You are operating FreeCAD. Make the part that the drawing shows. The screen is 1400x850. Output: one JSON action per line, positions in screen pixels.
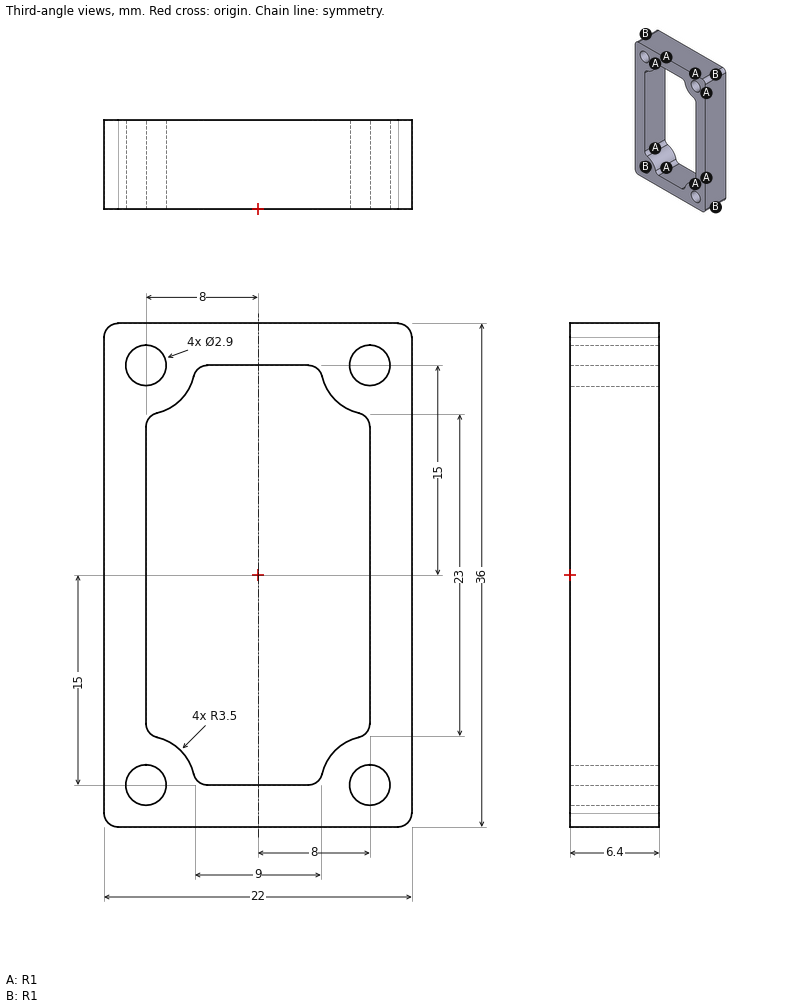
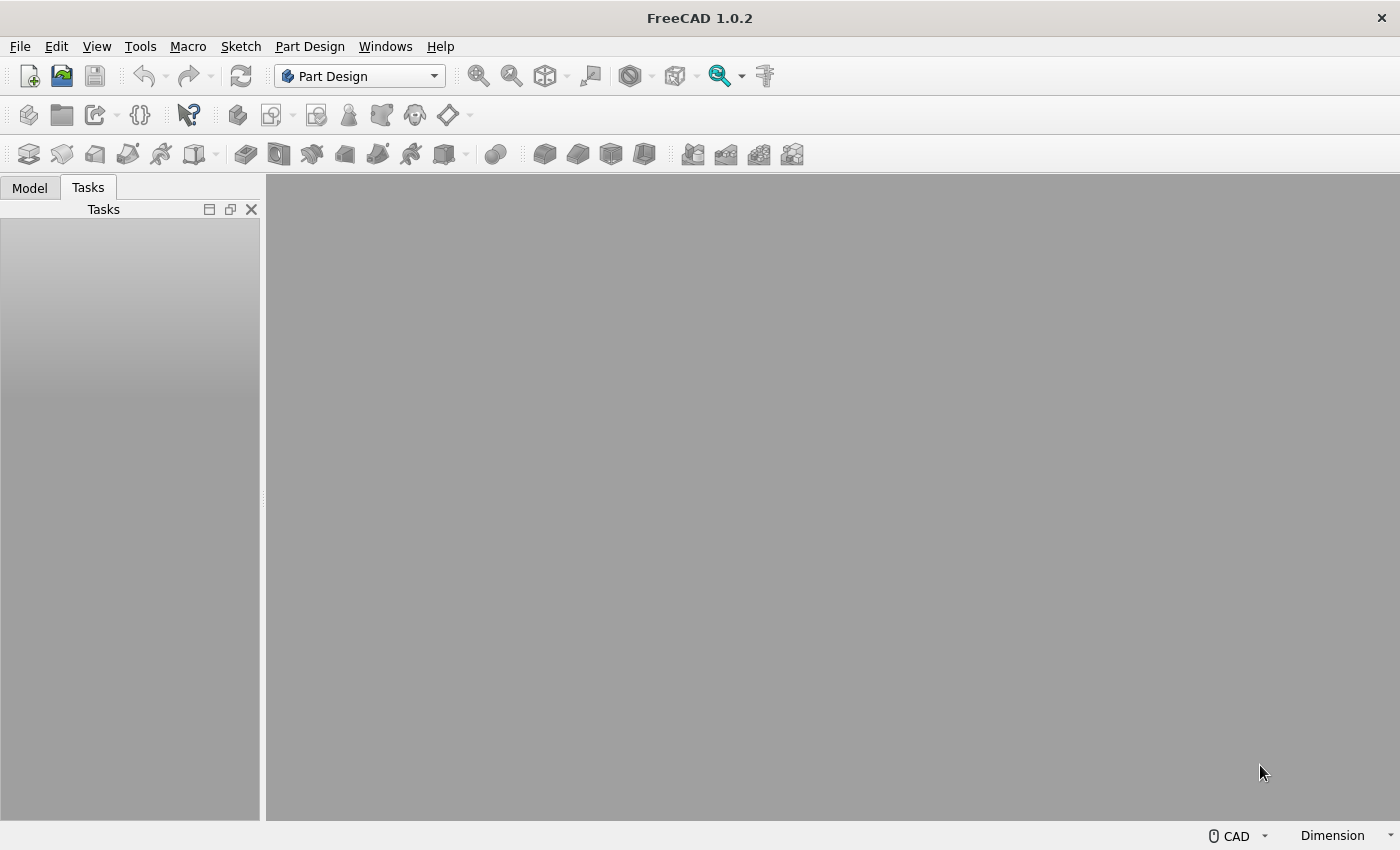
{"action": "left_click", "coordinate": [29, 76]}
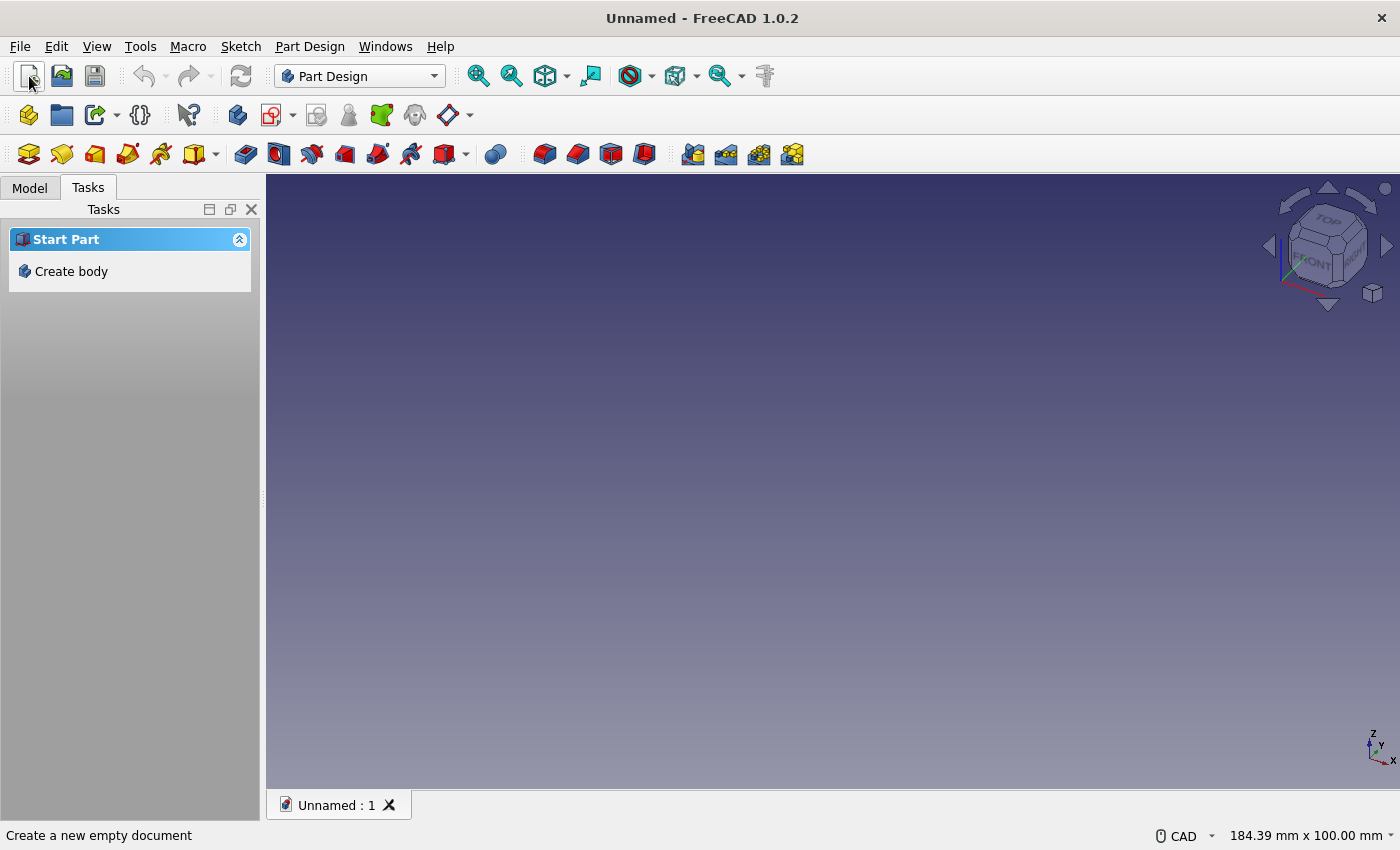
{"action": "left_click", "coordinate": [270, 116]}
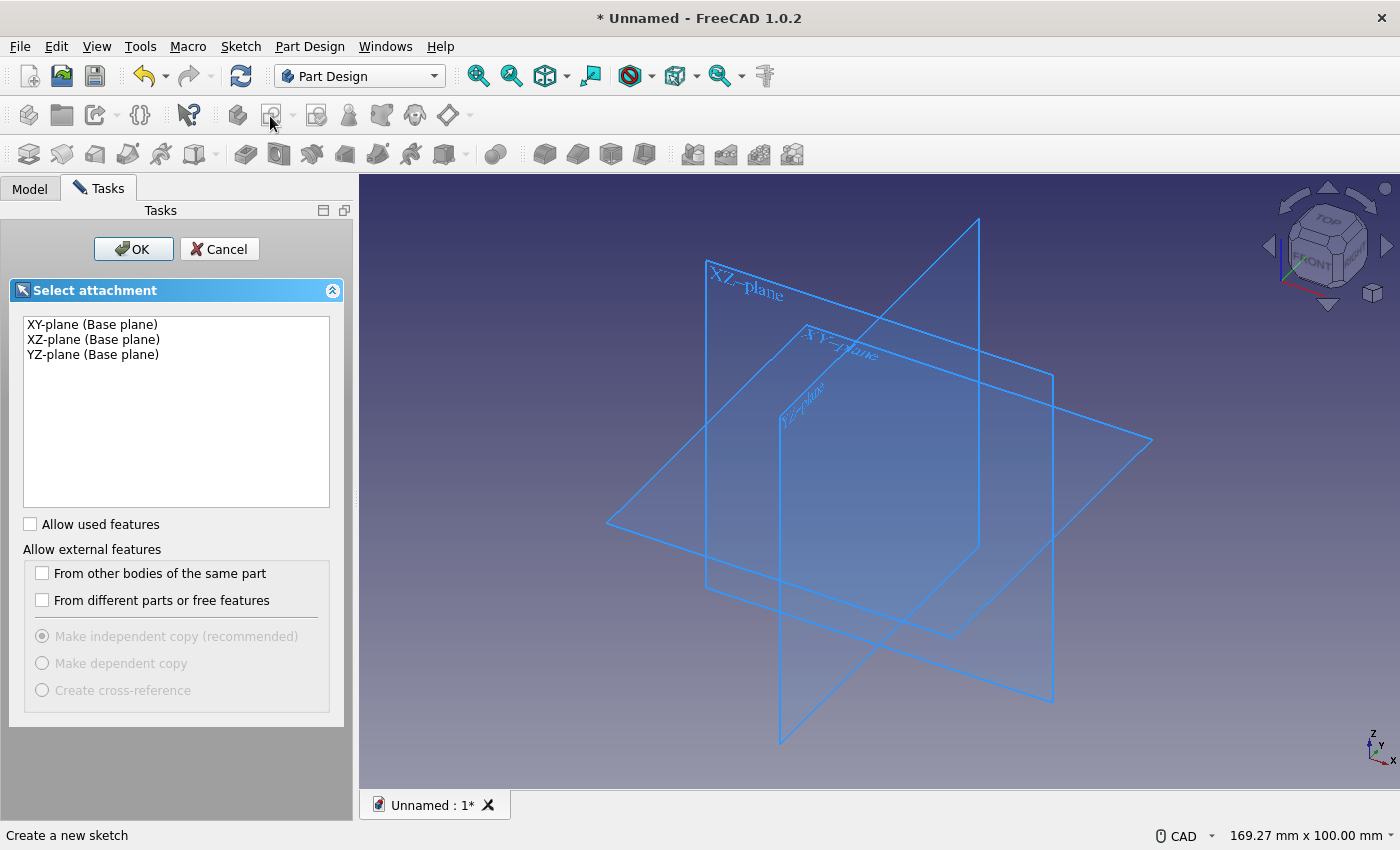
{"action": "left_click", "coordinate": [84, 340]}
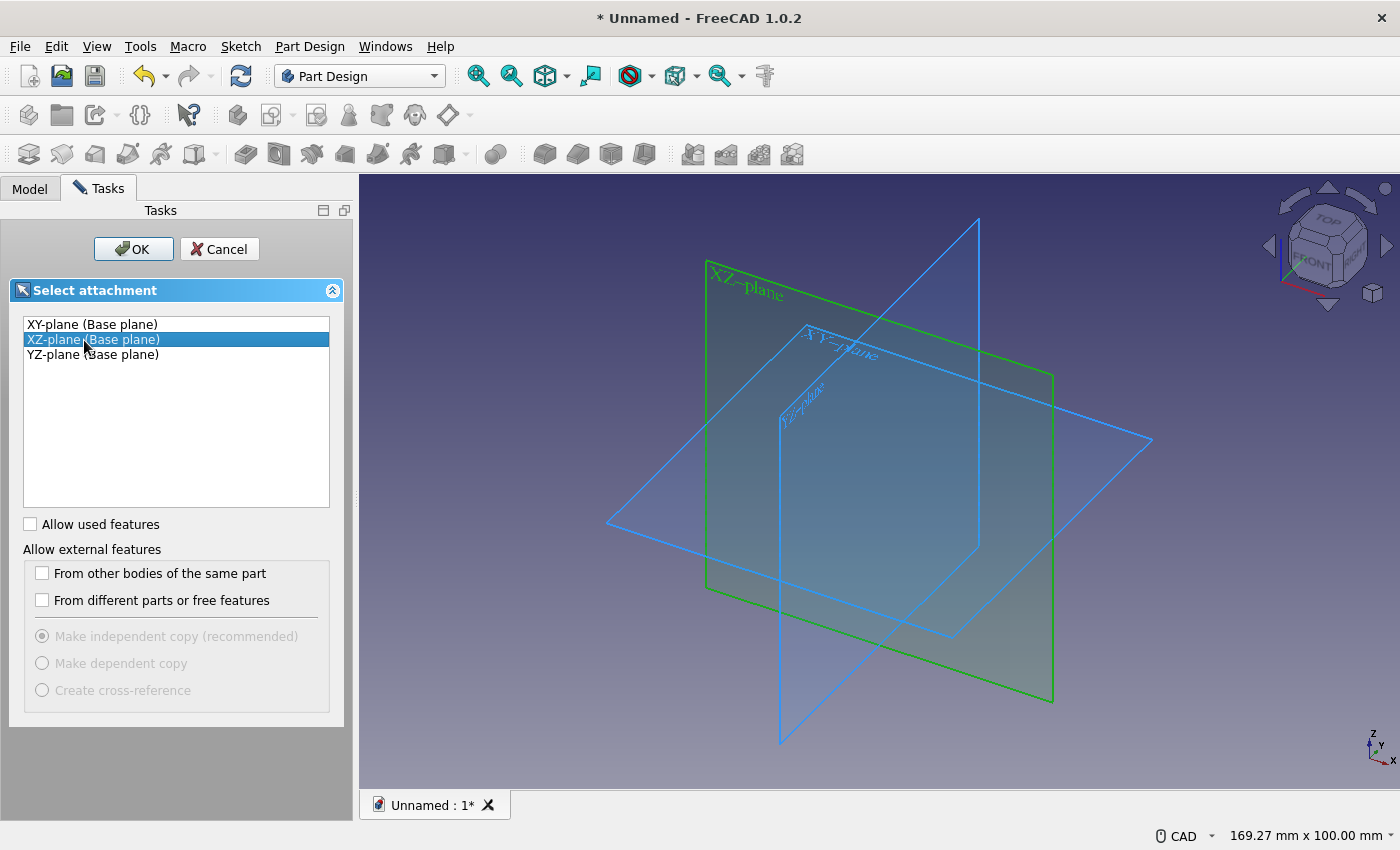
{"action": "left_click", "coordinate": [134, 249]}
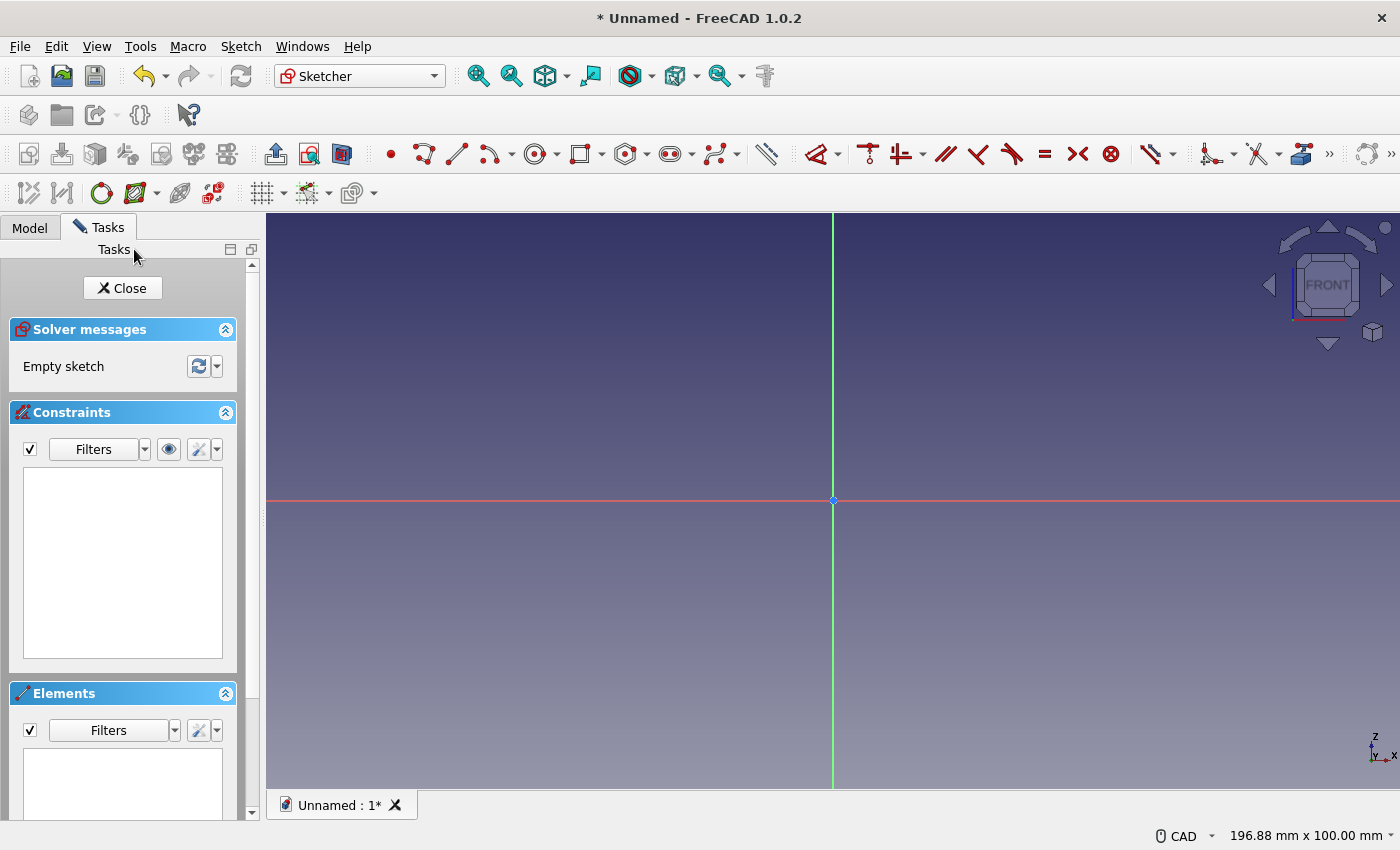
{"action": "scroll", "coordinate": [916, 501], "scroll_direction": "up", "scroll_amount": 3}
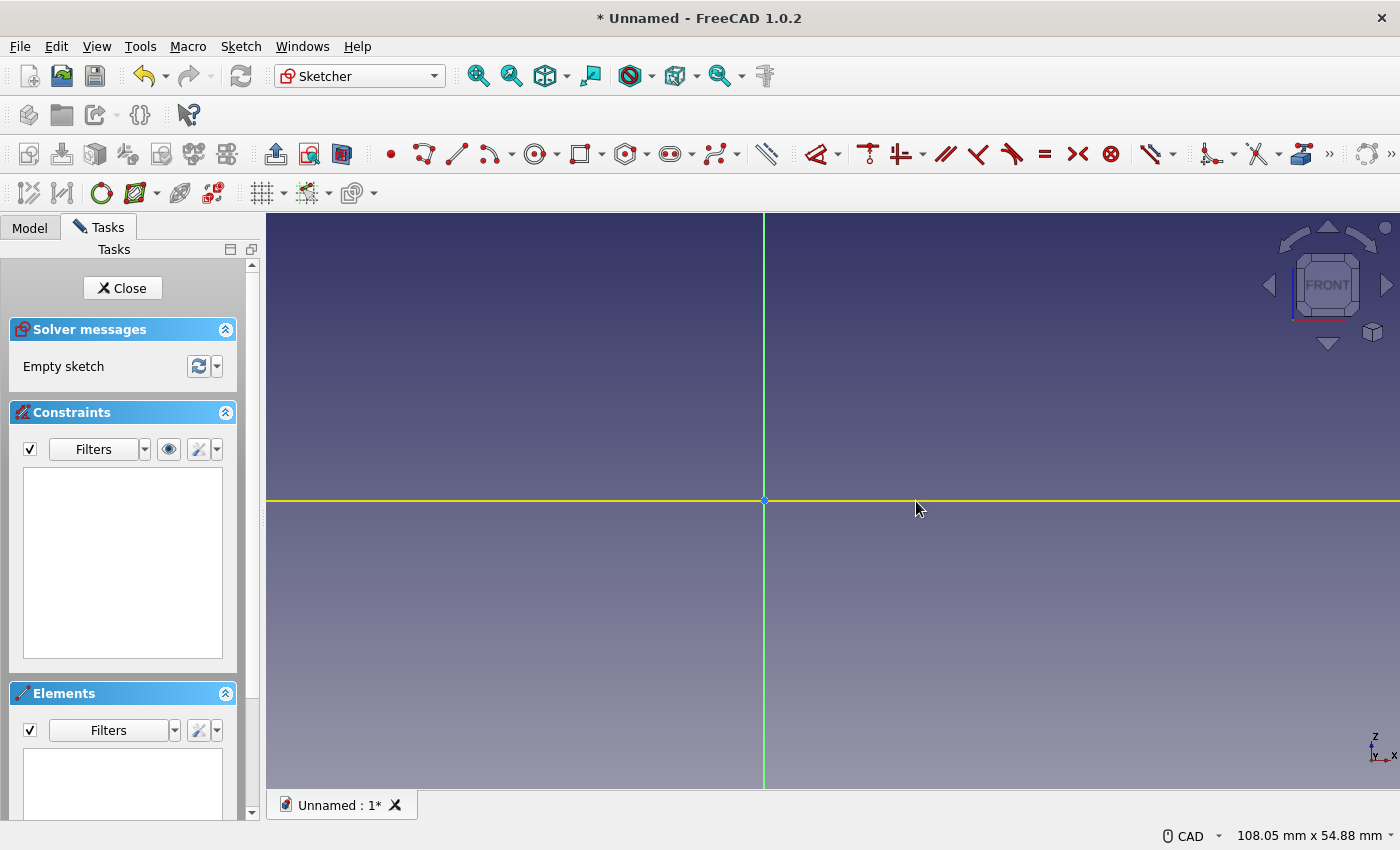
{"action": "key", "text": "g v"}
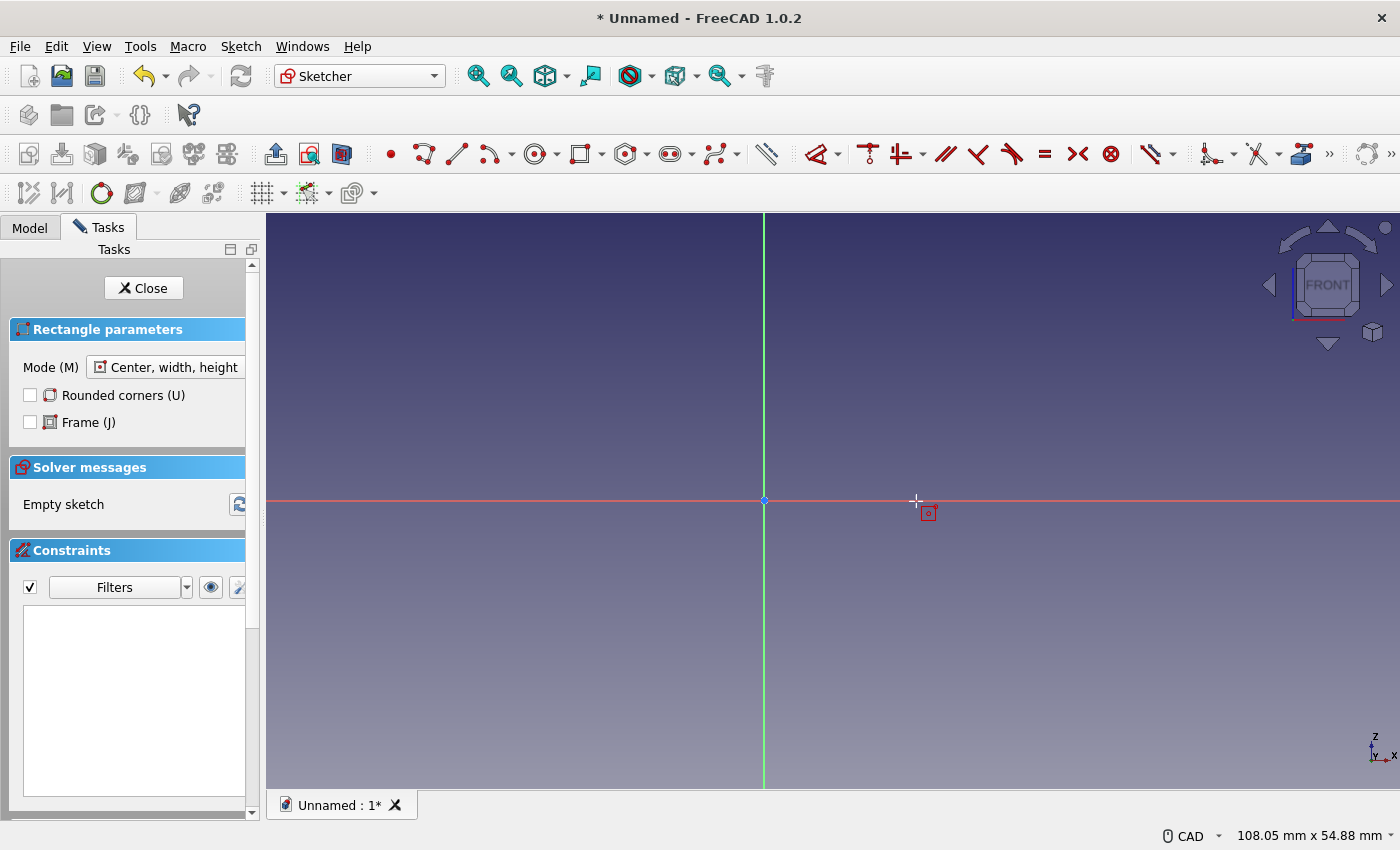
{"action": "left_click", "coordinate": [764, 501]}
{"action": "mouse_move", "coordinate": [880, 312]}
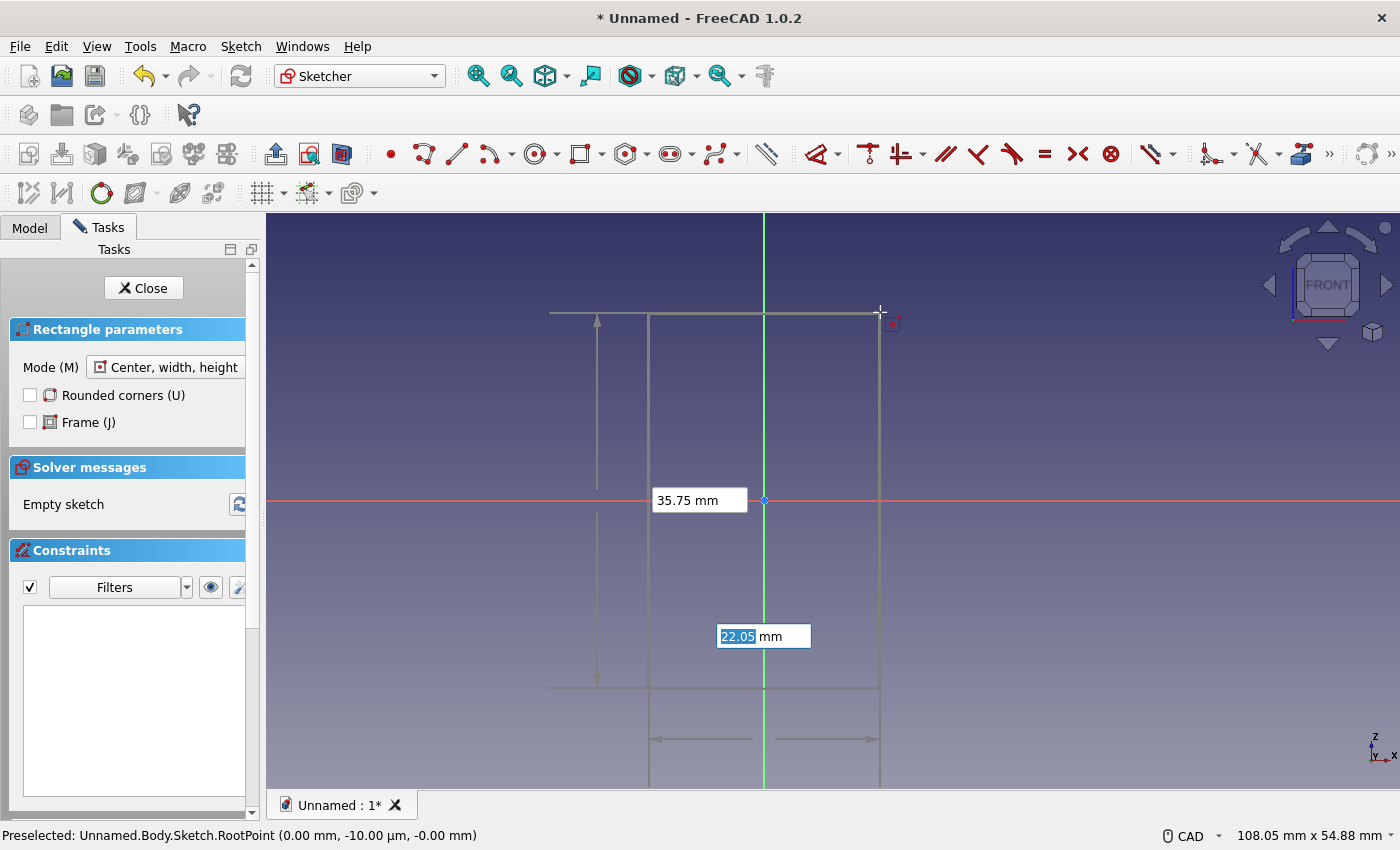
{"action": "type", "text": "22"}
{"action": "key", "text": "Tab"}
{"action": "type", "text": "36"}
{"action": "key", "text": "Return"}